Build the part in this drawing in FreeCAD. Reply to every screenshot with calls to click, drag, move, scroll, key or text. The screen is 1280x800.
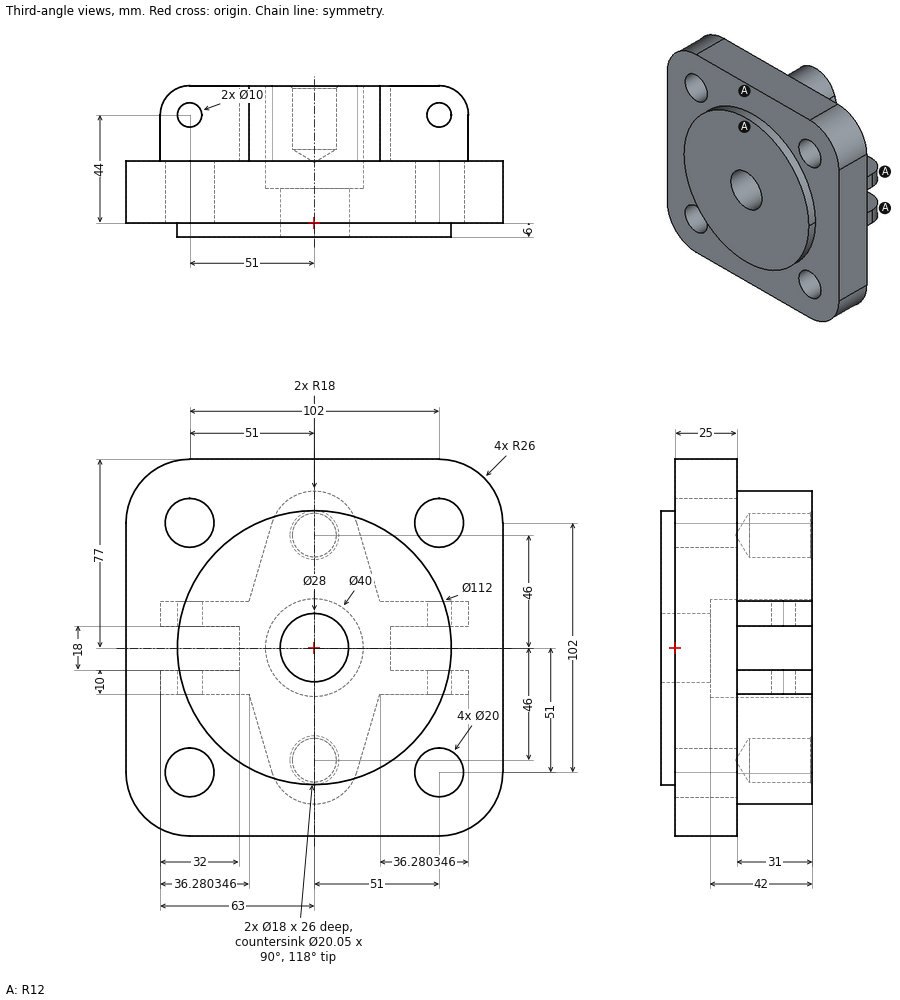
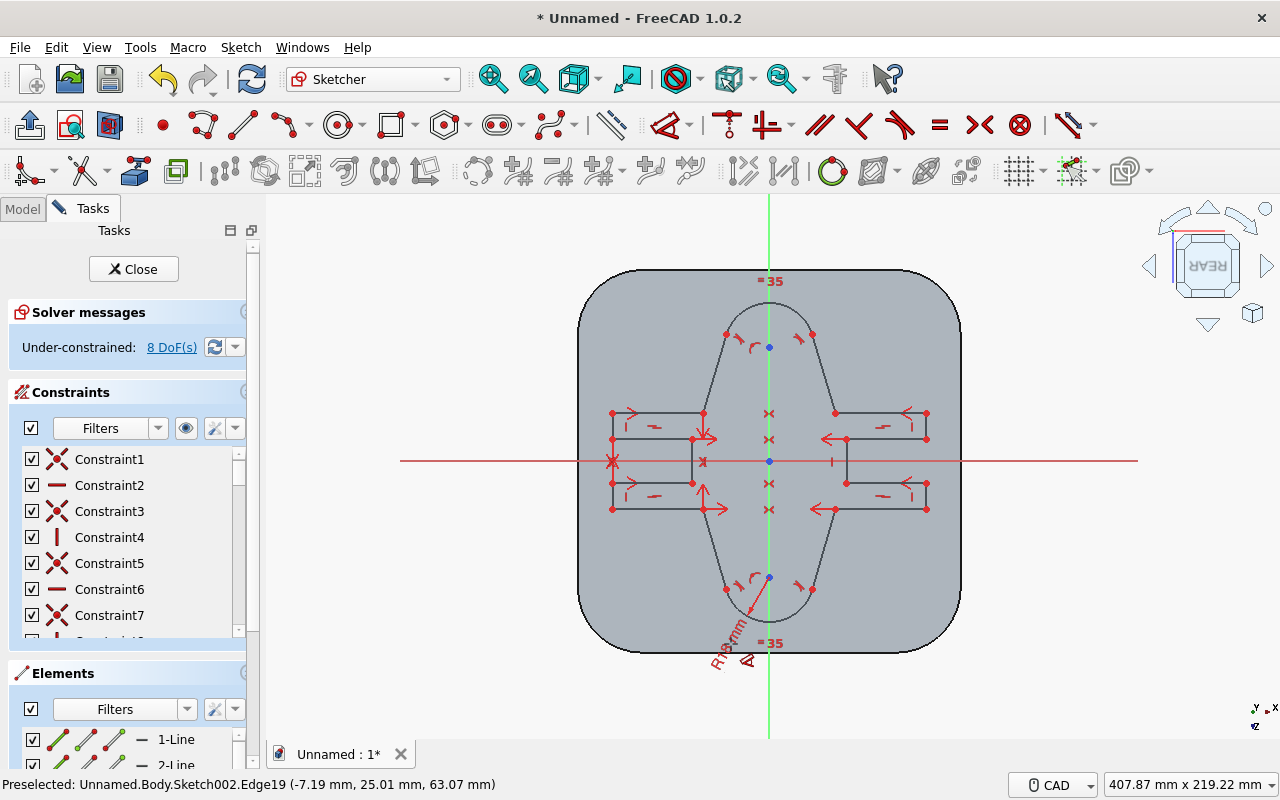
scroll(613, 424, up, 3)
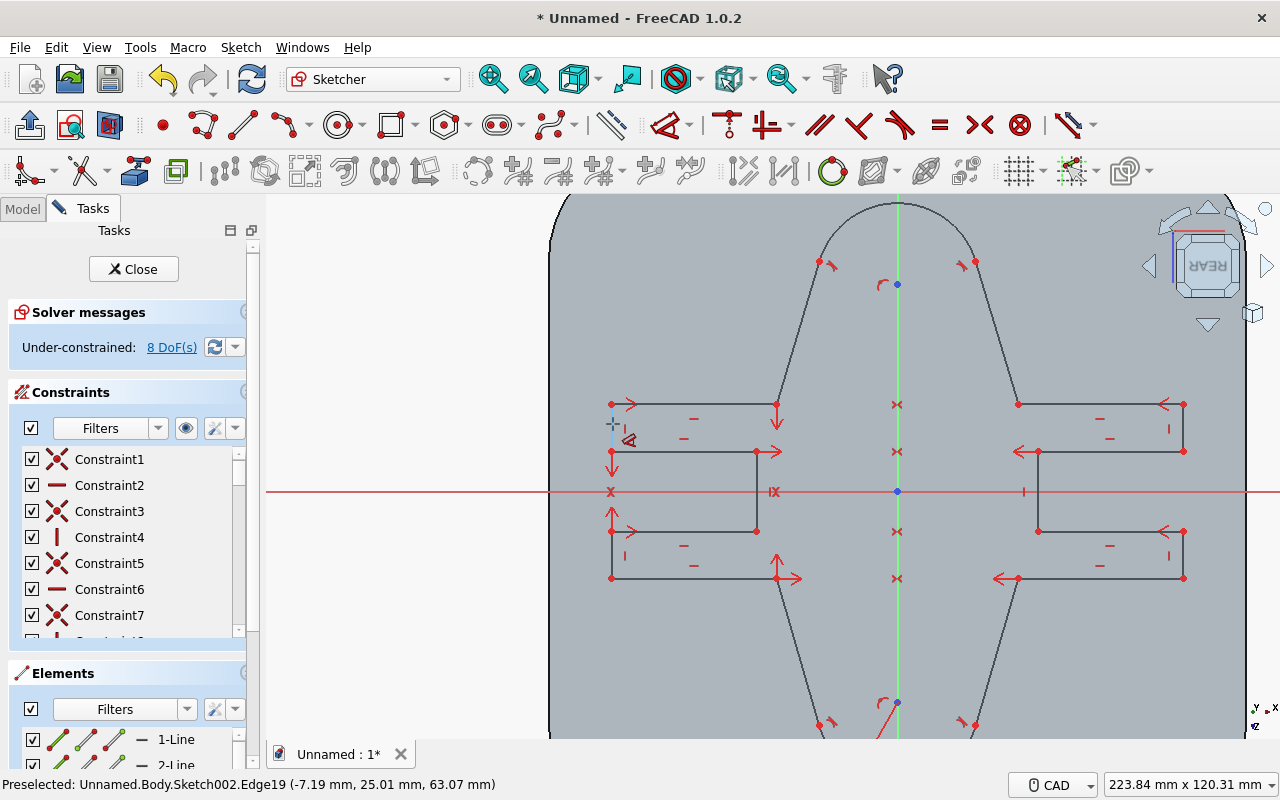
click(612, 423)
click(578, 428)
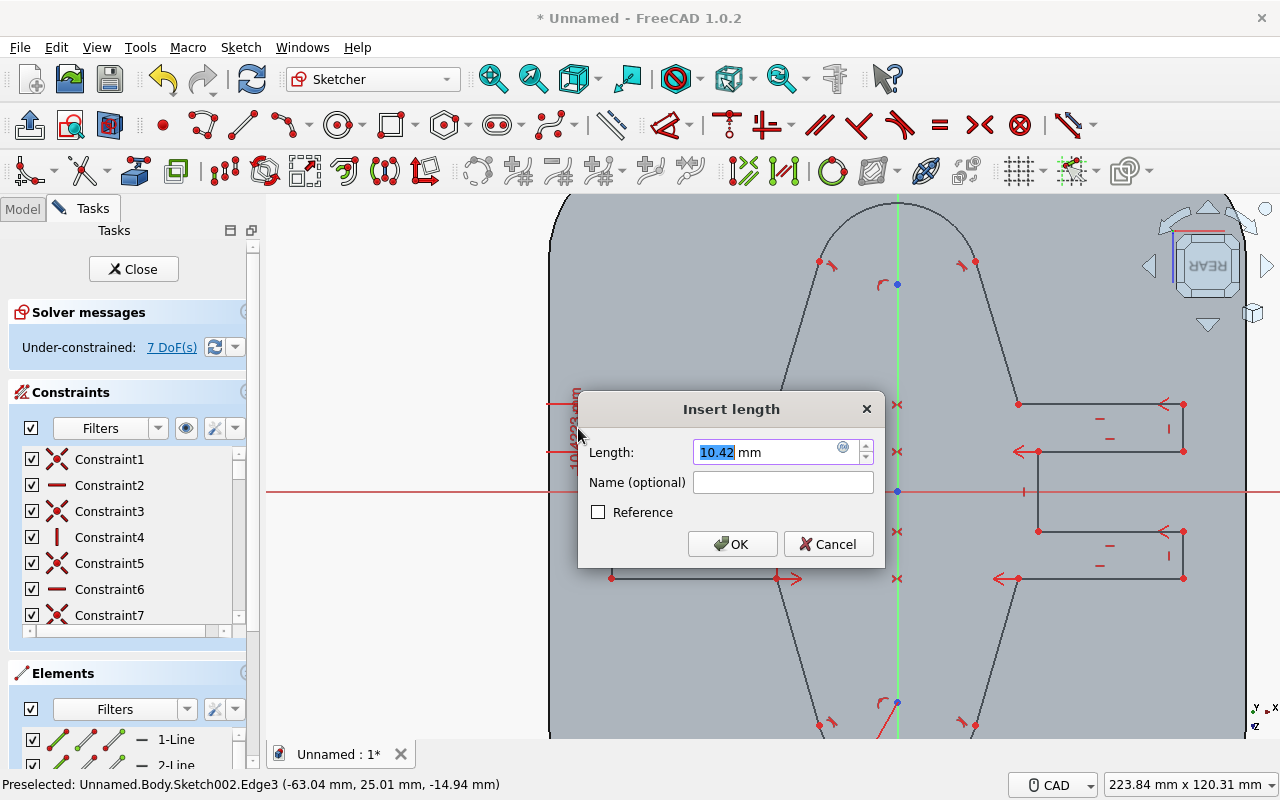
text(10)
key(Return)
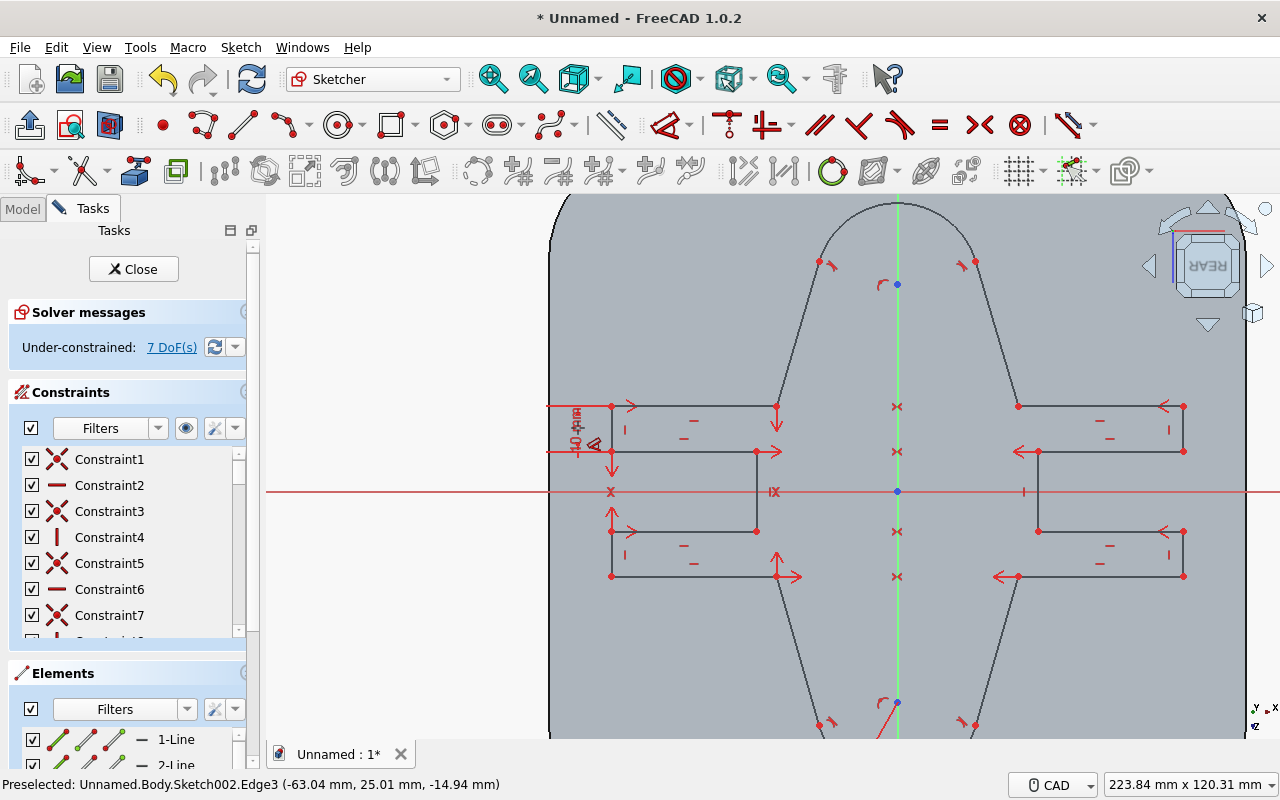
click(655, 452)
click(684, 510)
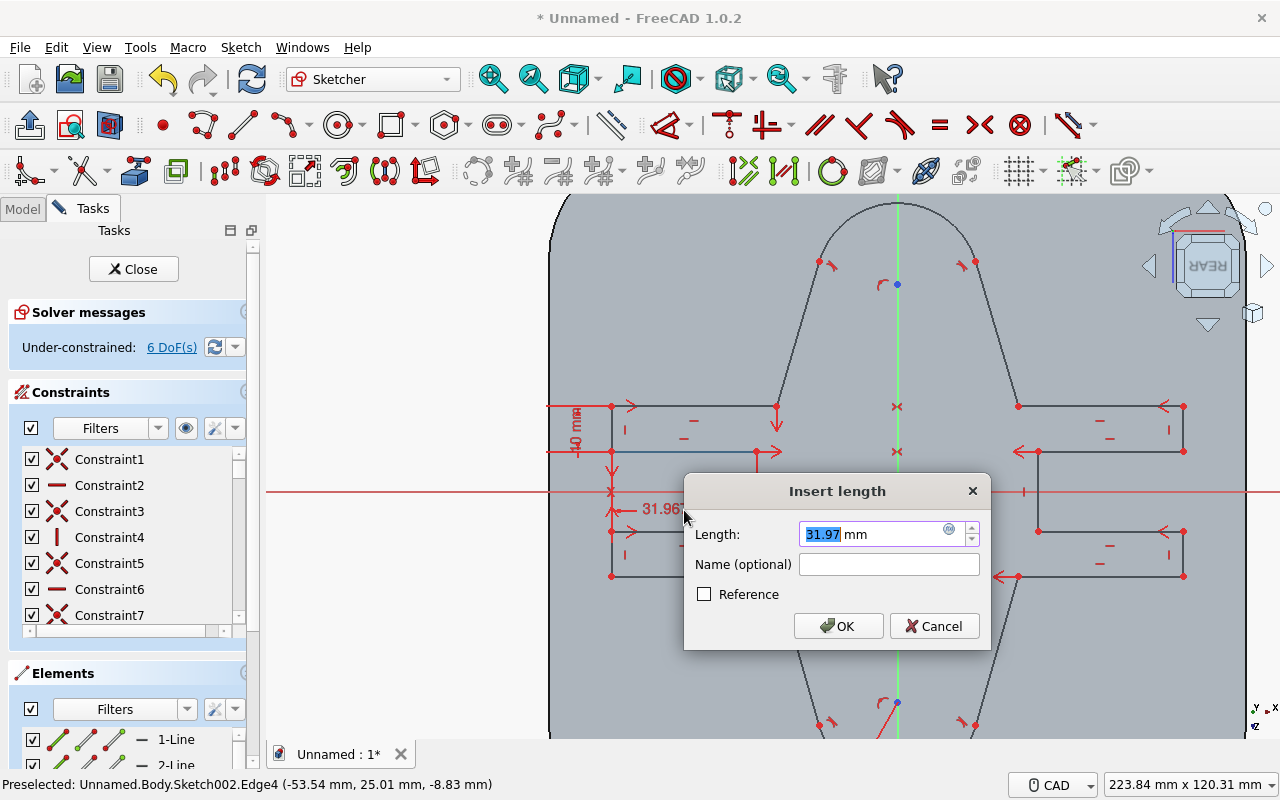
text(32)
key(Return)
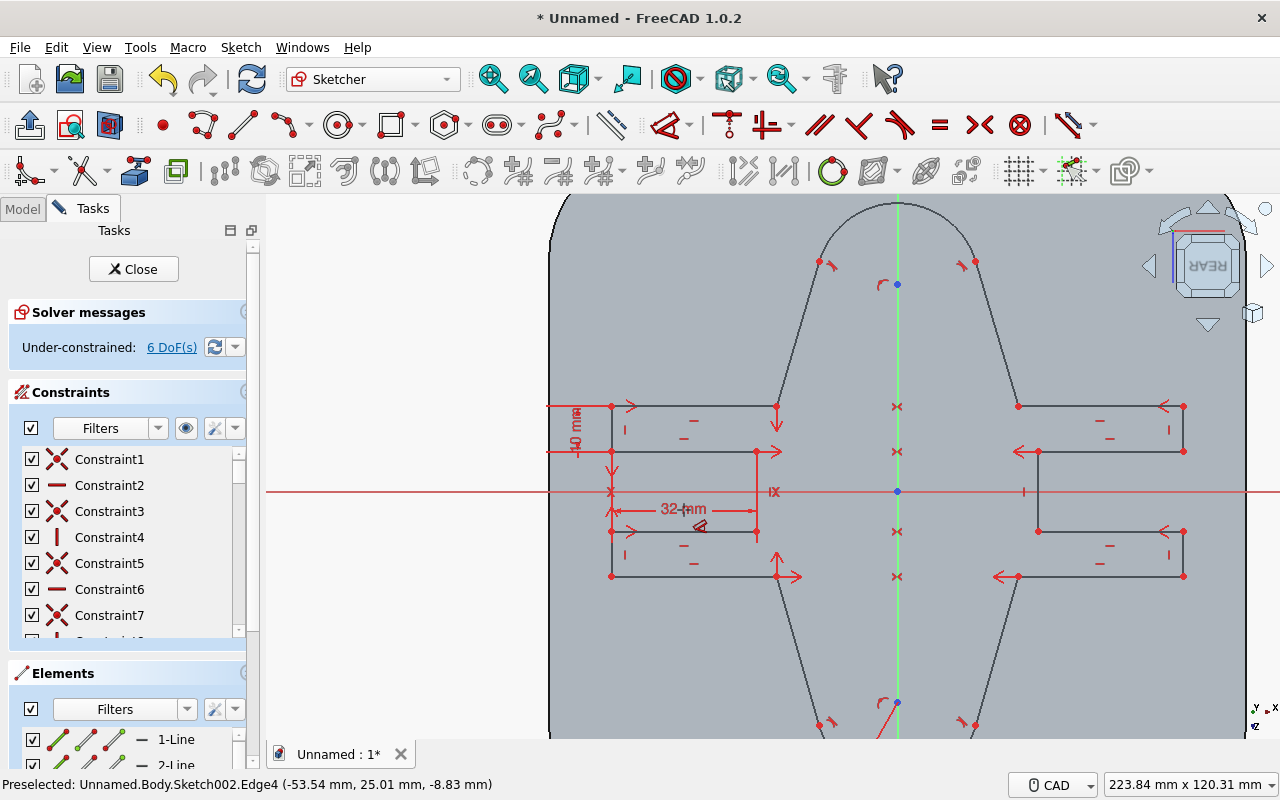
click(757, 476)
click(723, 473)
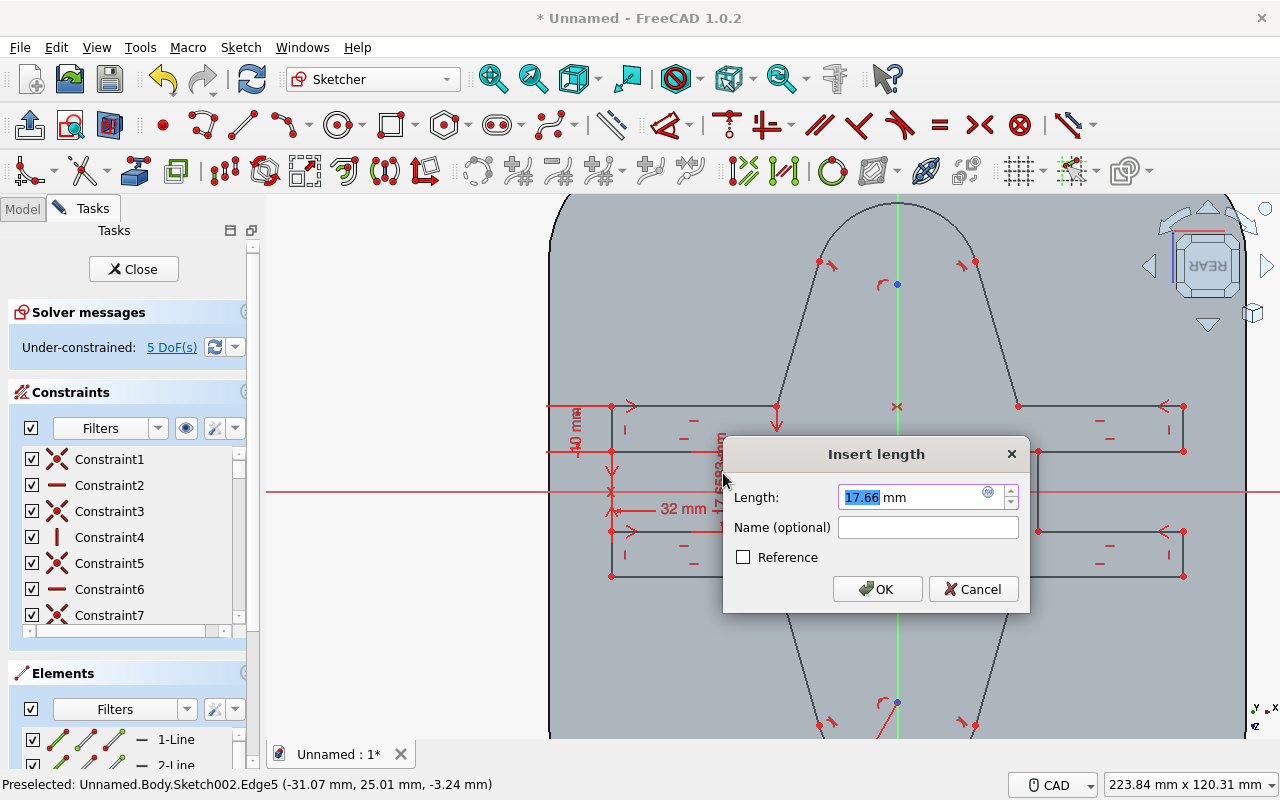
text(18)
key(Return)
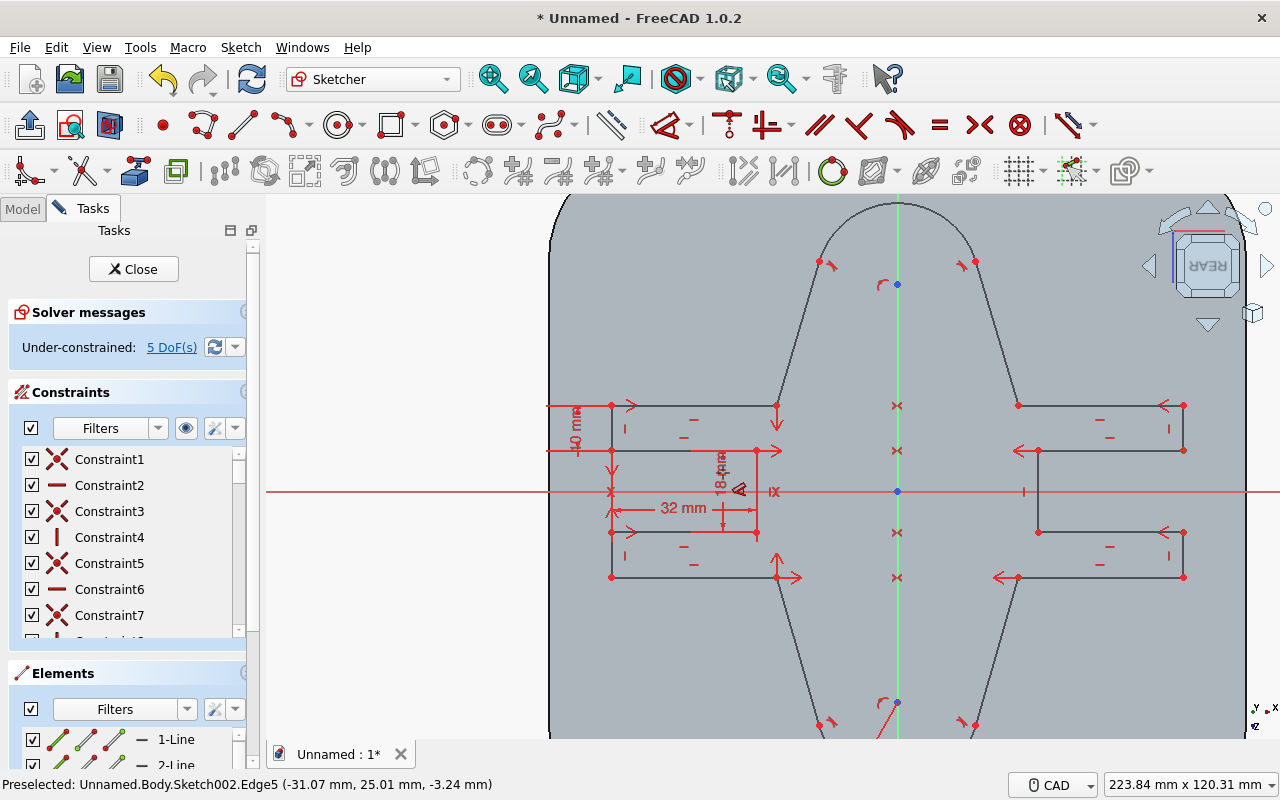
click(612, 406)
click(755, 372)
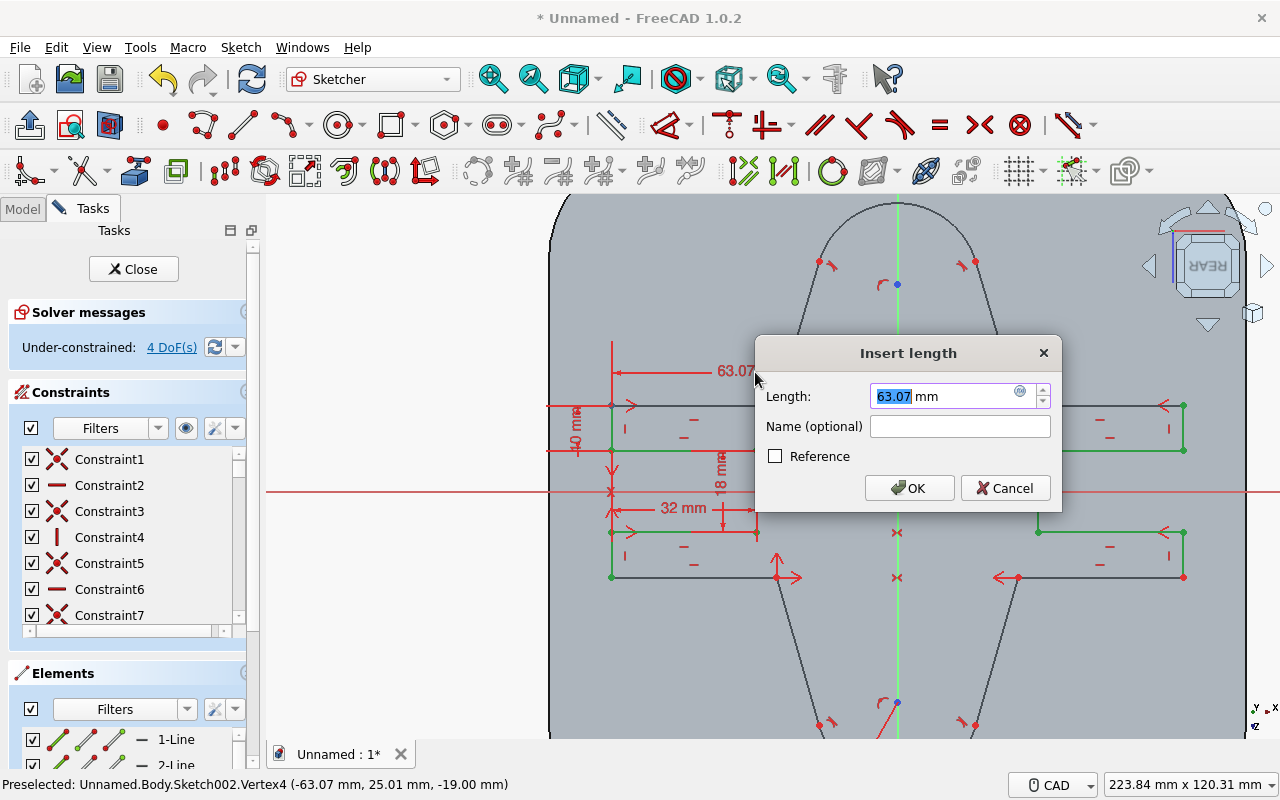
text(63)
key(Return)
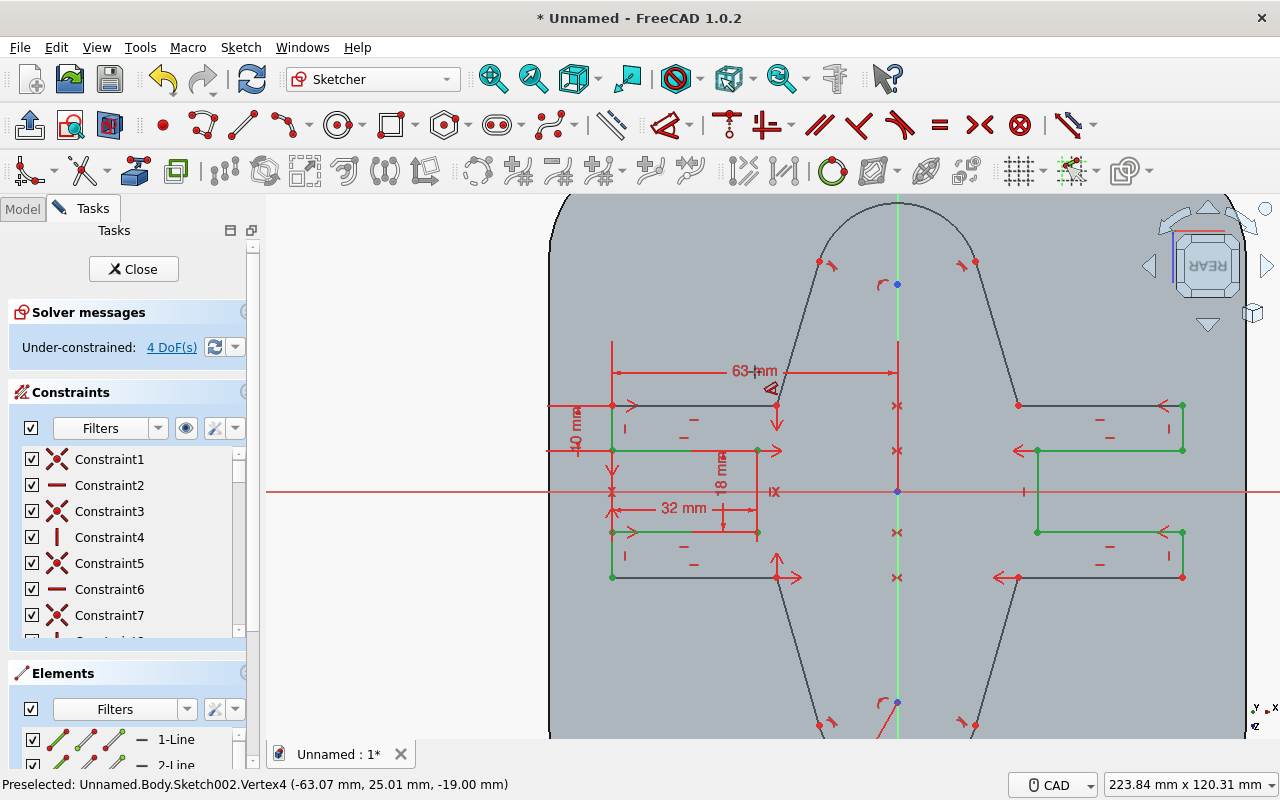
click(898, 703)
click(932, 597)